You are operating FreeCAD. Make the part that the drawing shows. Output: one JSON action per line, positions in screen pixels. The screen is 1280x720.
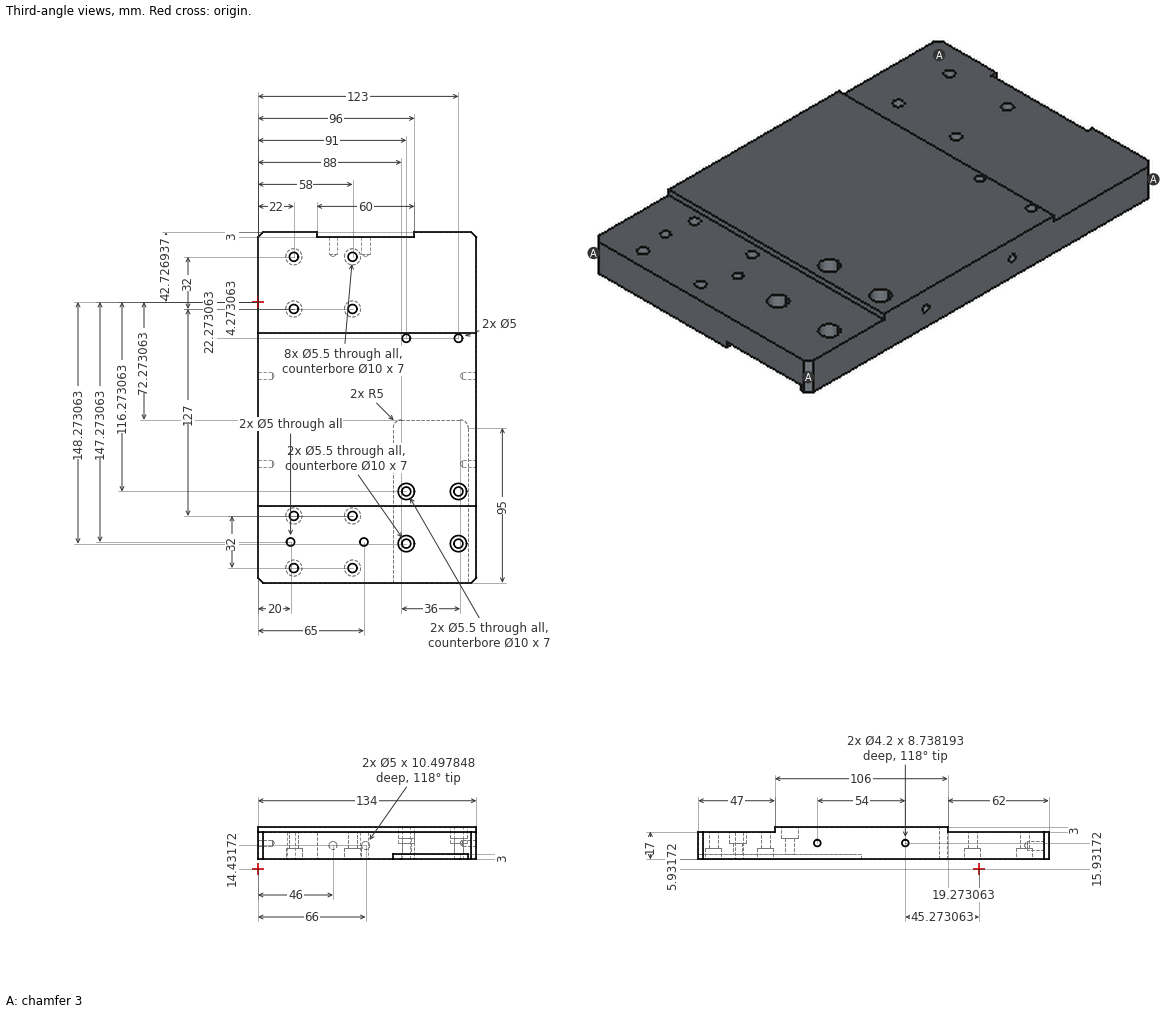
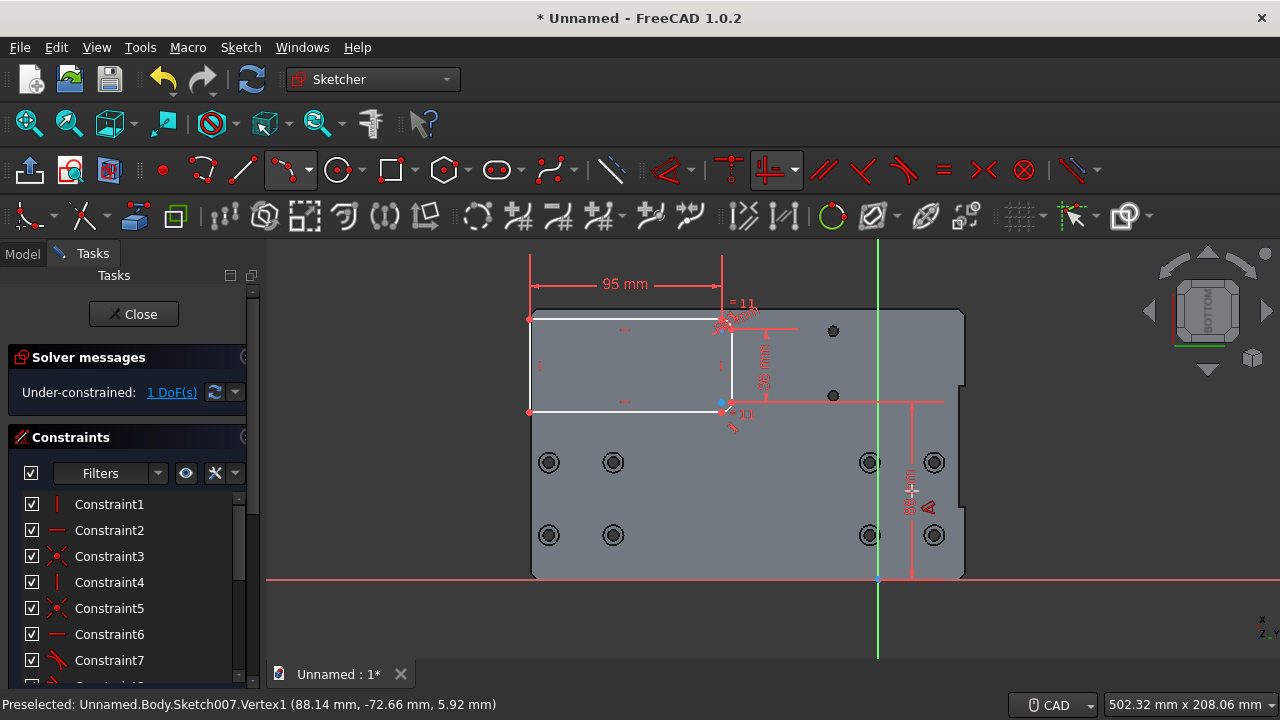
{"action": "left_click", "coordinate": [732, 402]}
{"action": "left_click", "coordinate": [805, 614]}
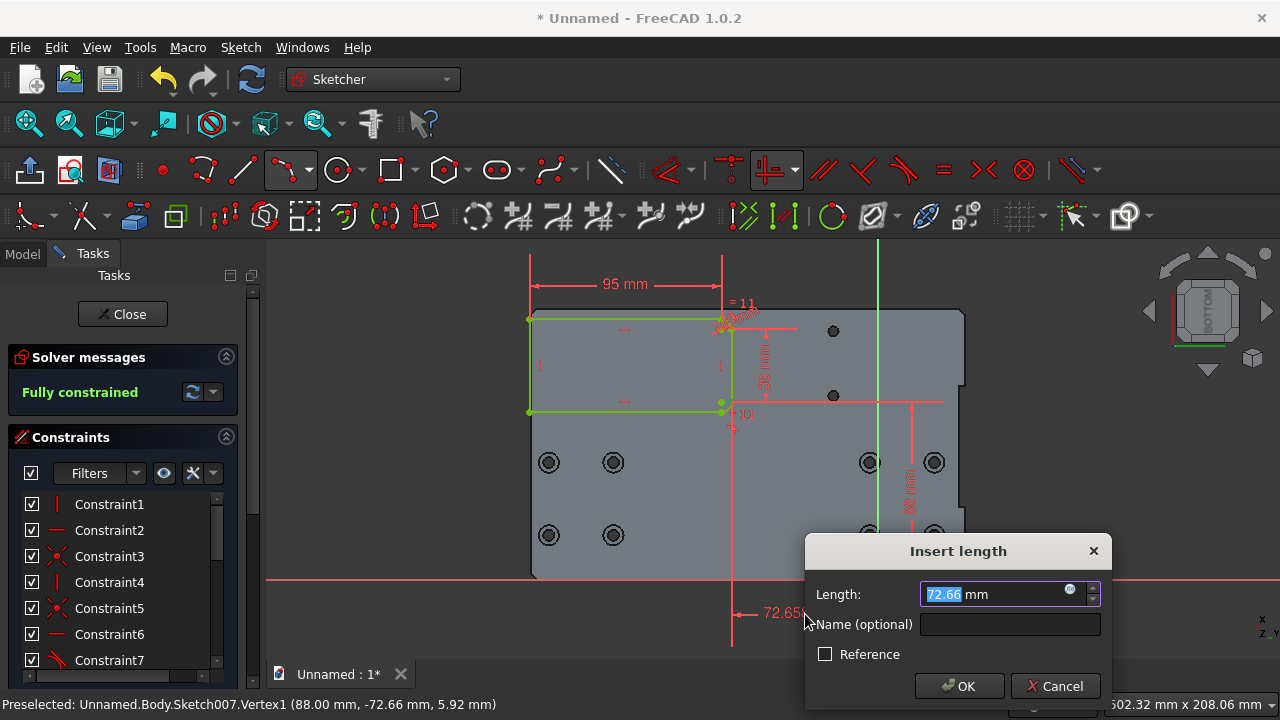
{"action": "type", "text": "72.273063"}
{"action": "key", "text": "Return"}
{"action": "key", "text": "Escape"}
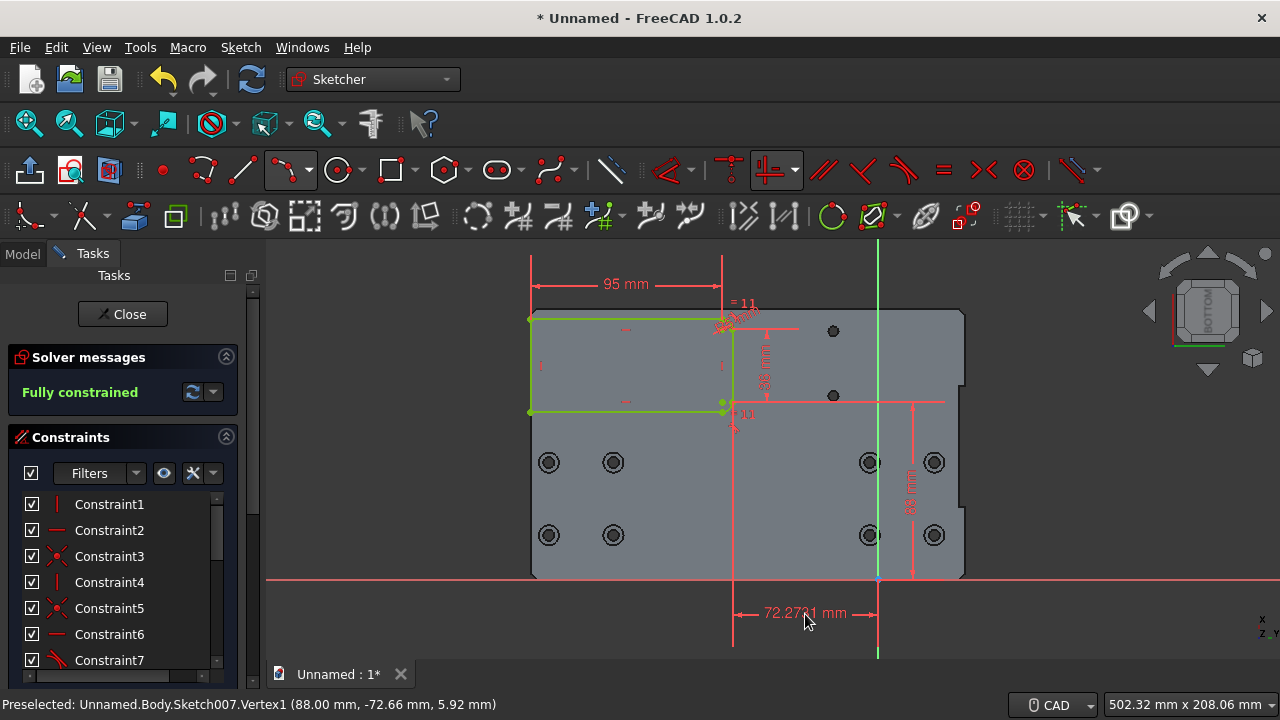
{"action": "left_click", "coordinate": [123, 314]}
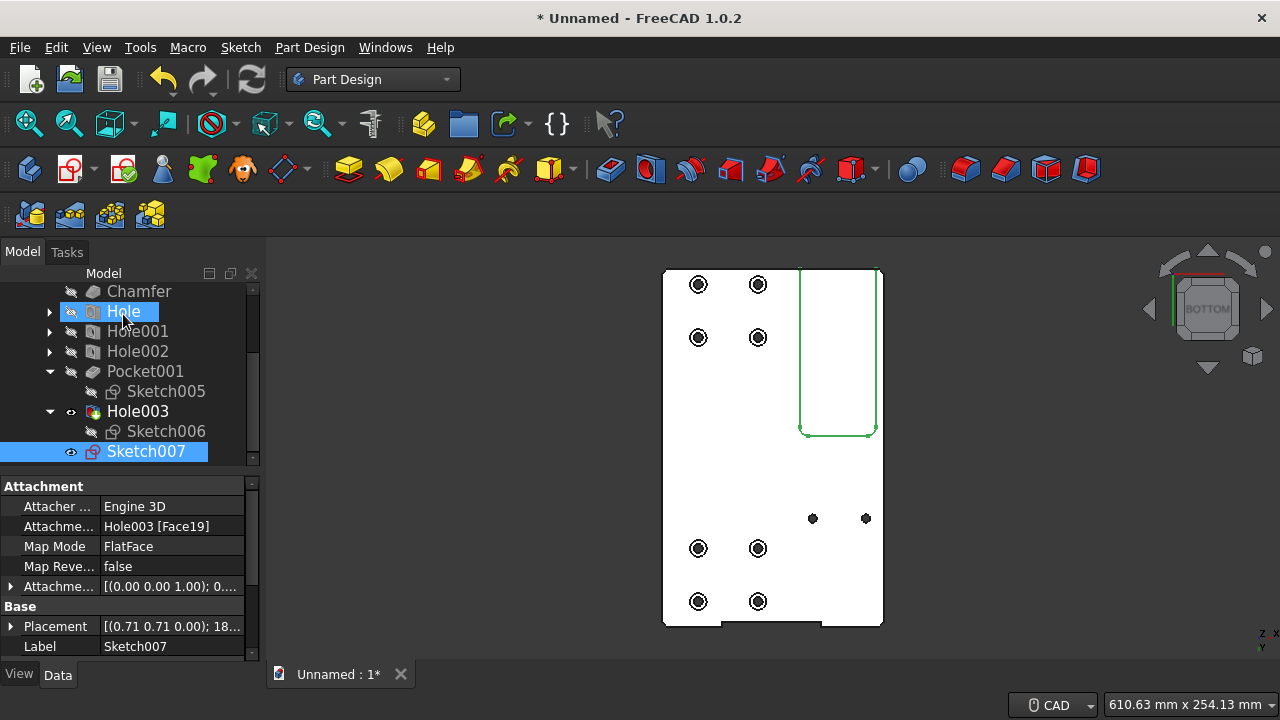
{"action": "left_click", "coordinate": [612, 170]}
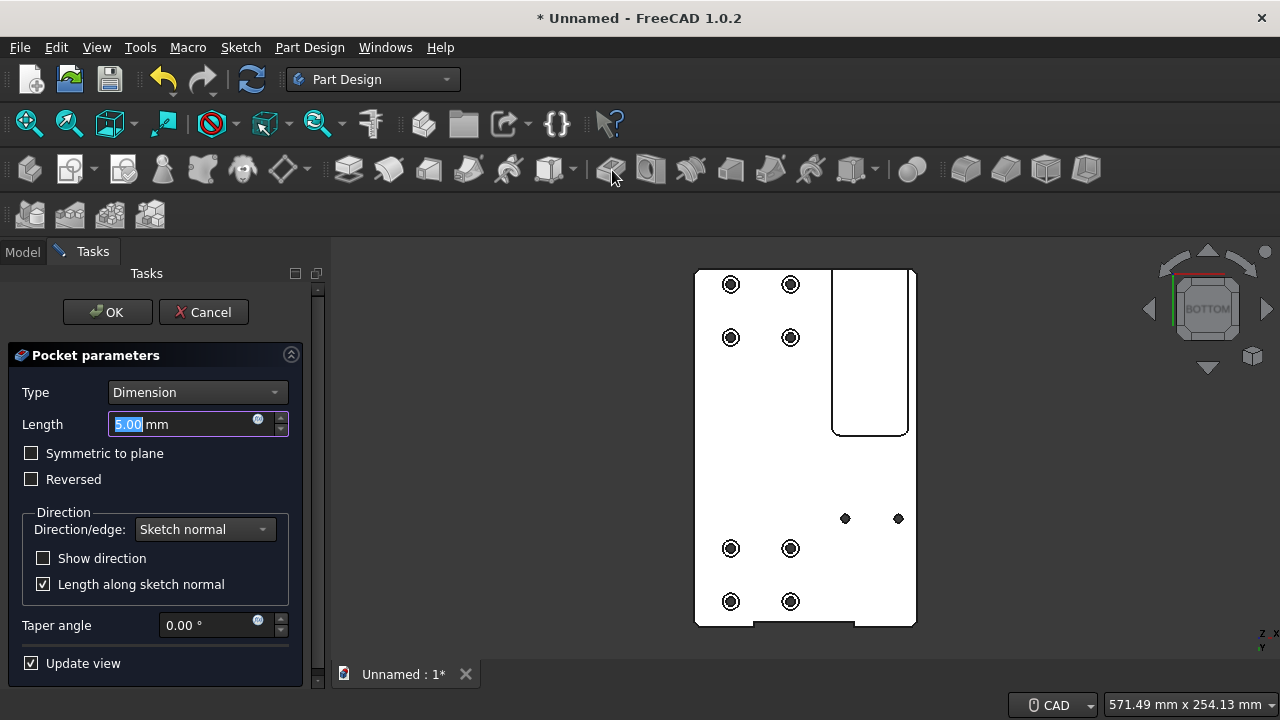
{"action": "type", "text": "3"}
{"action": "key", "text": "Tab"}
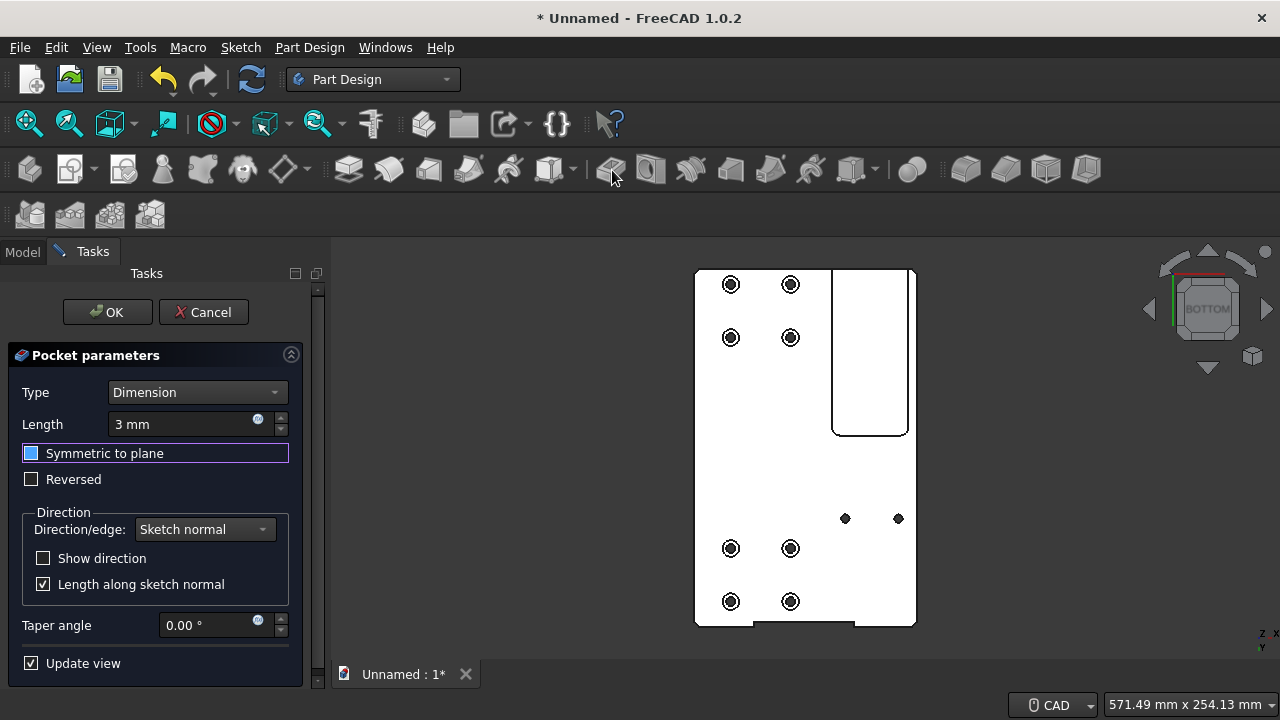
{"action": "left_click", "coordinate": [108, 312]}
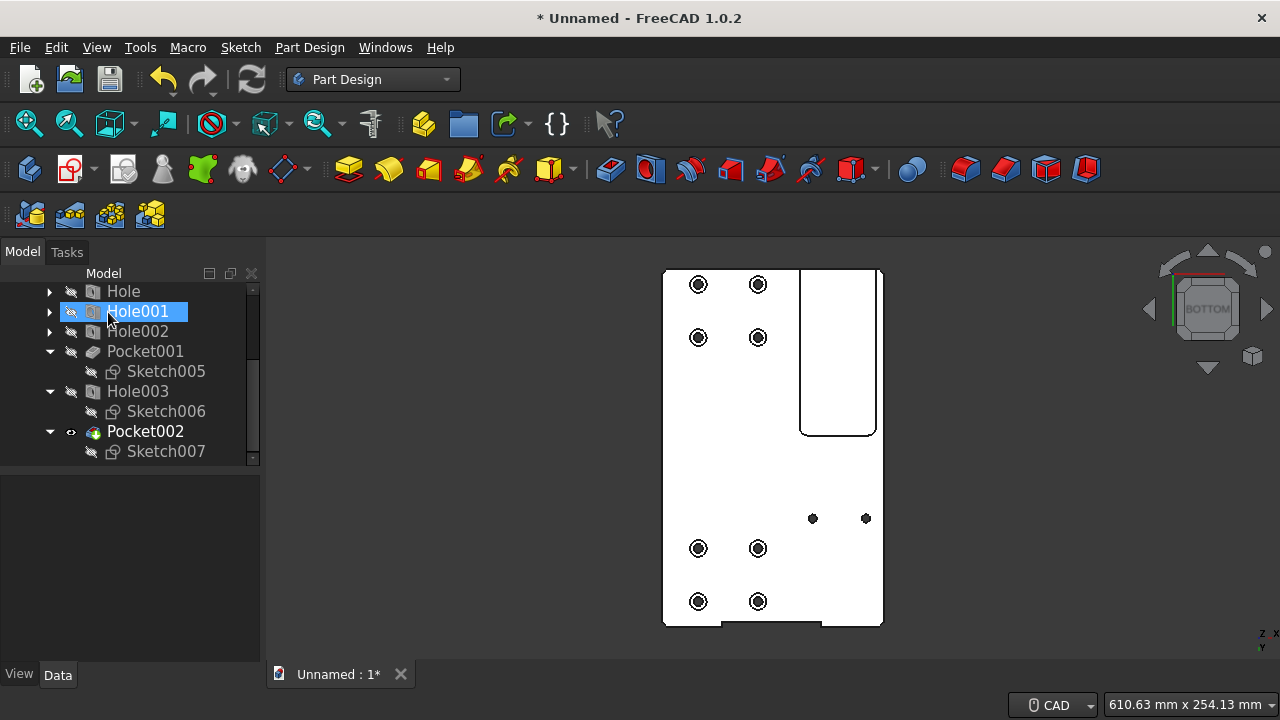
{"action": "key", "text": "0"}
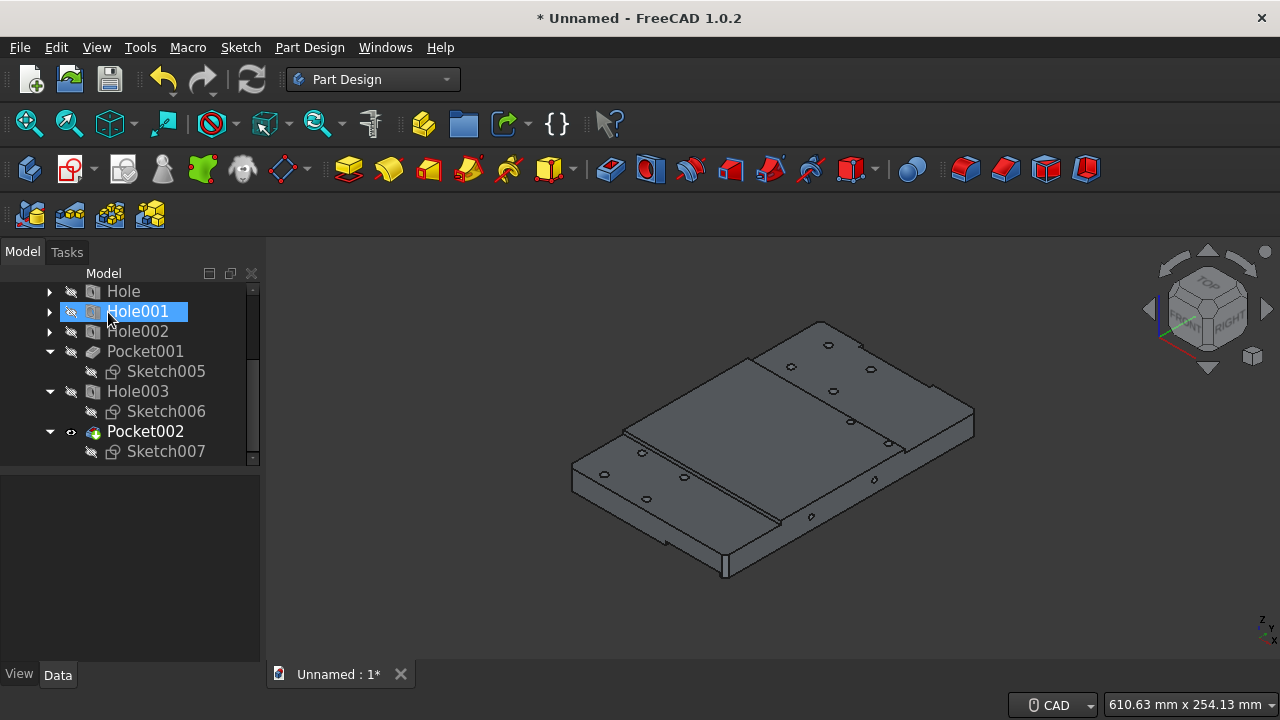
{"action": "left_click", "coordinate": [764, 439]}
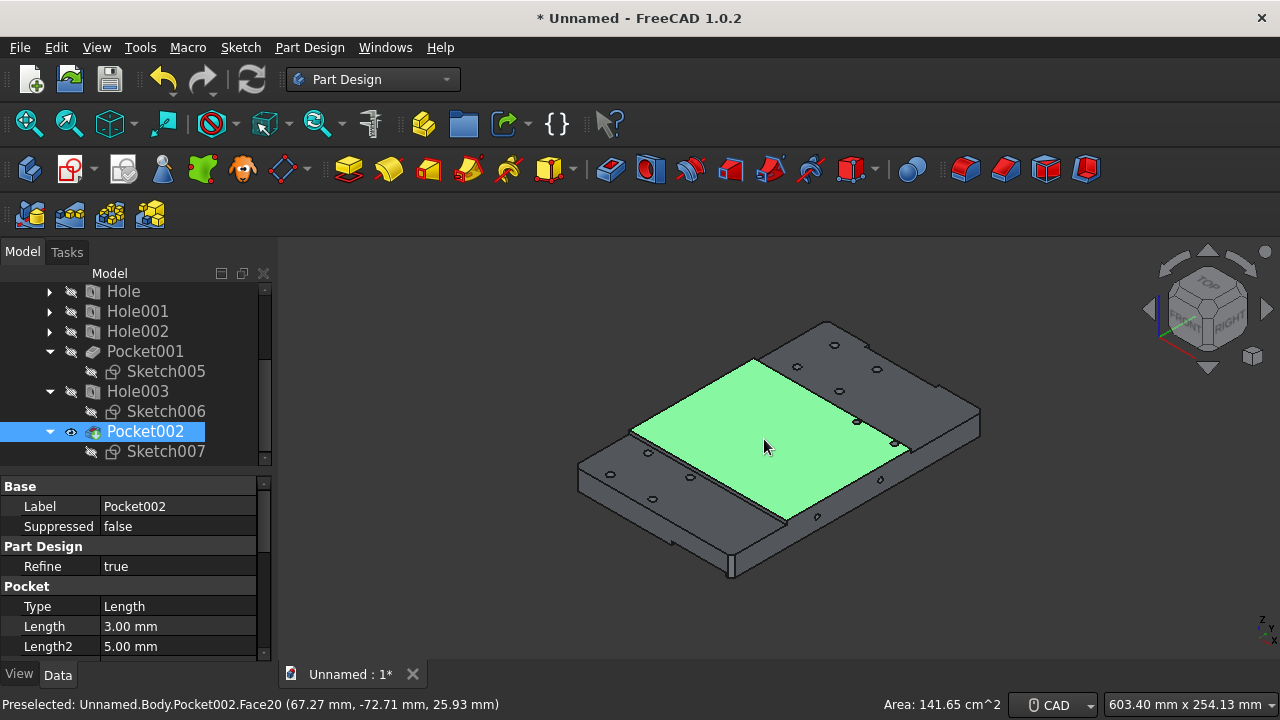
{"action": "left_click", "coordinate": [70, 170]}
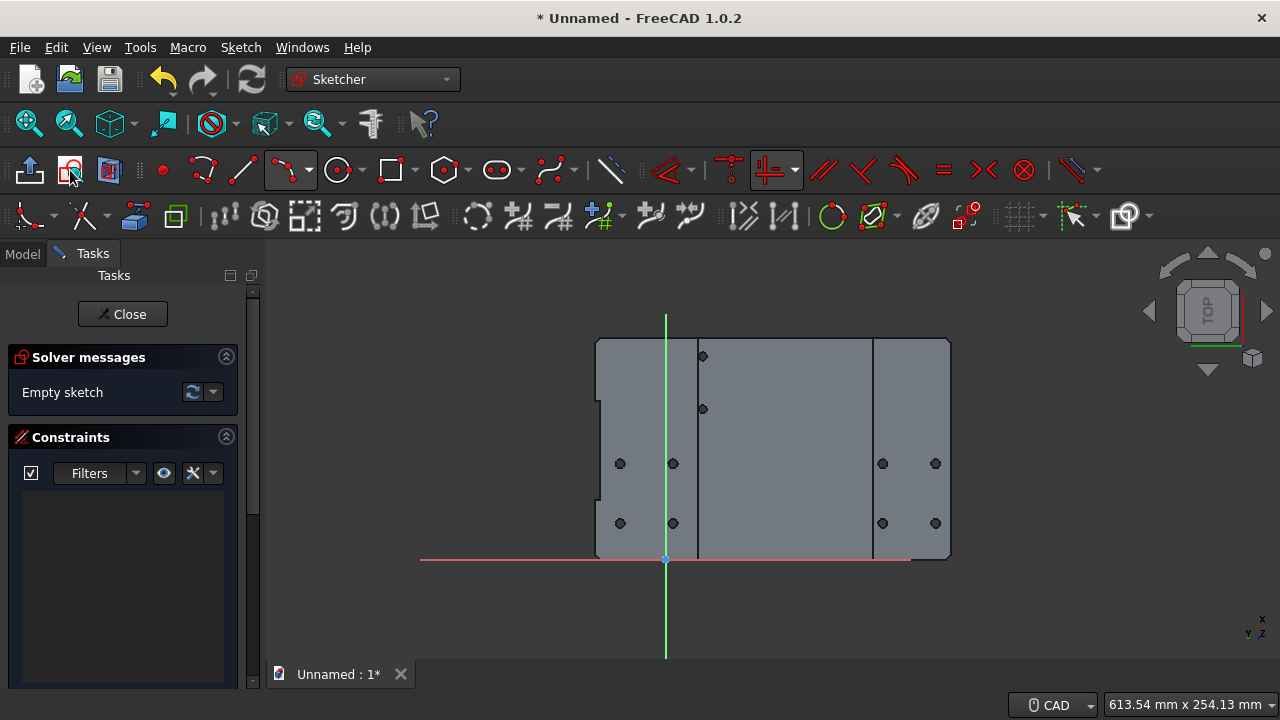
{"action": "scroll", "coordinate": [908, 361], "scroll_direction": "up", "scroll_amount": 7}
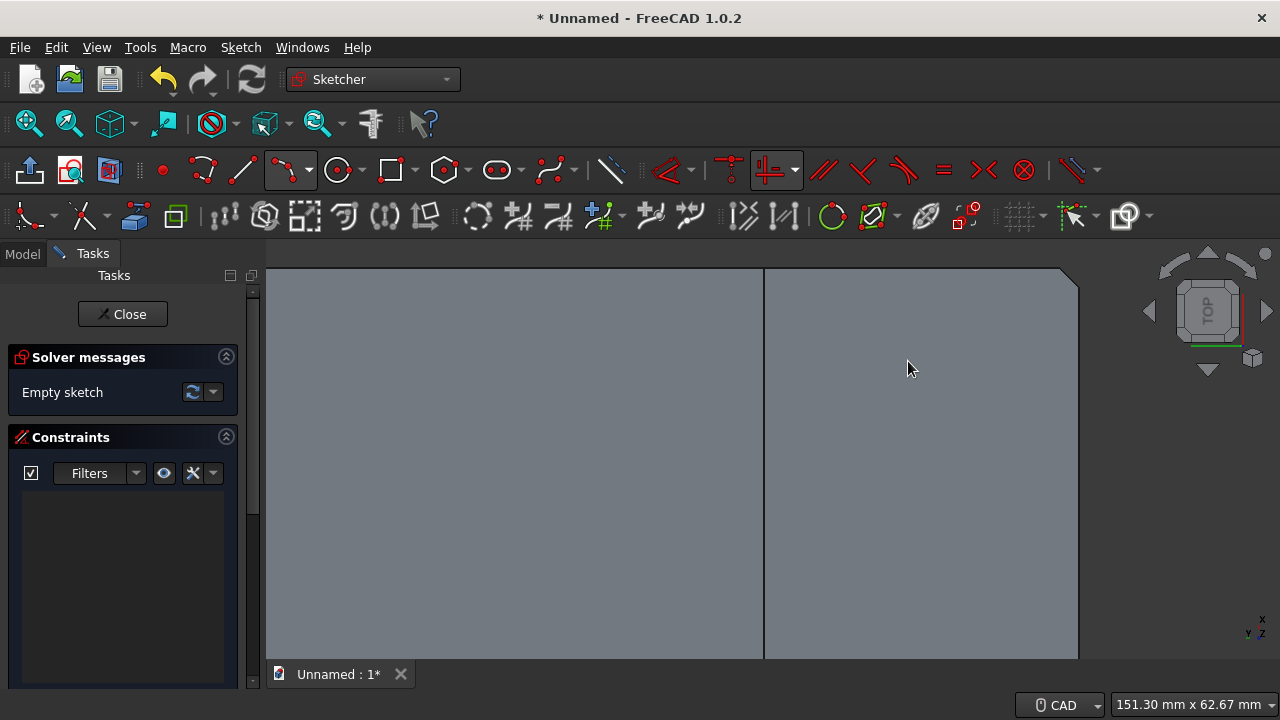
{"action": "left_click", "coordinate": [338, 170]}